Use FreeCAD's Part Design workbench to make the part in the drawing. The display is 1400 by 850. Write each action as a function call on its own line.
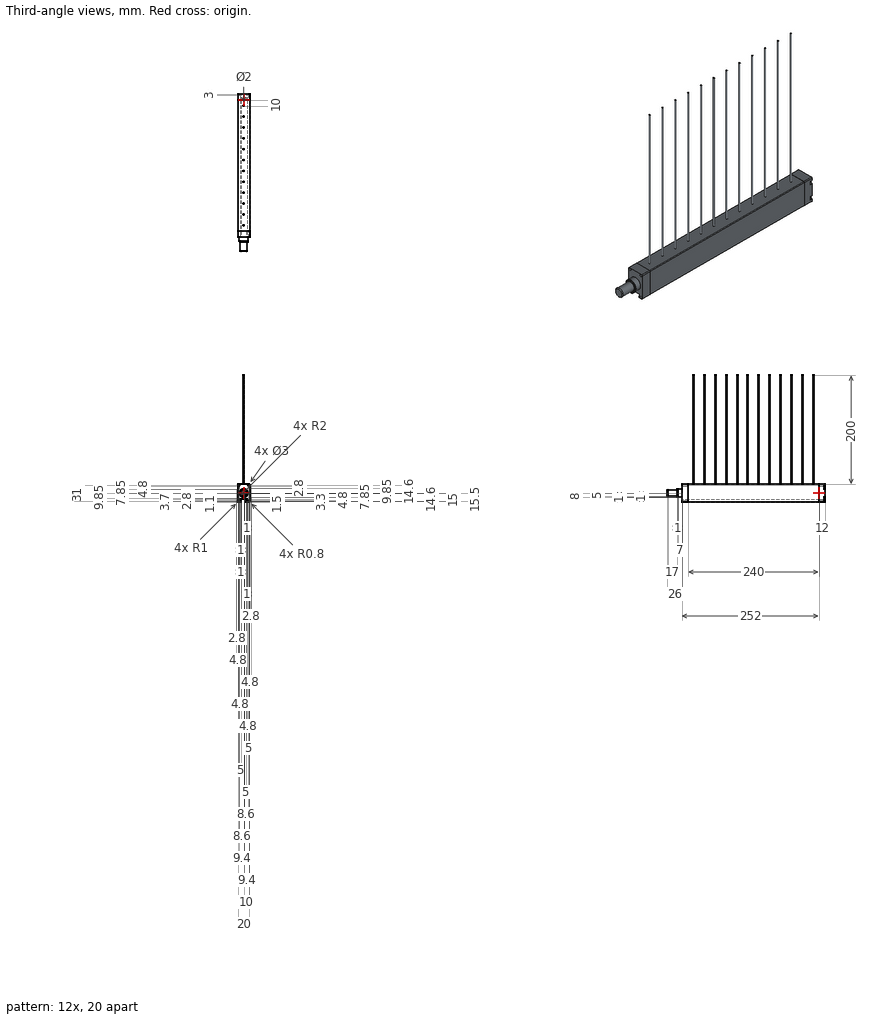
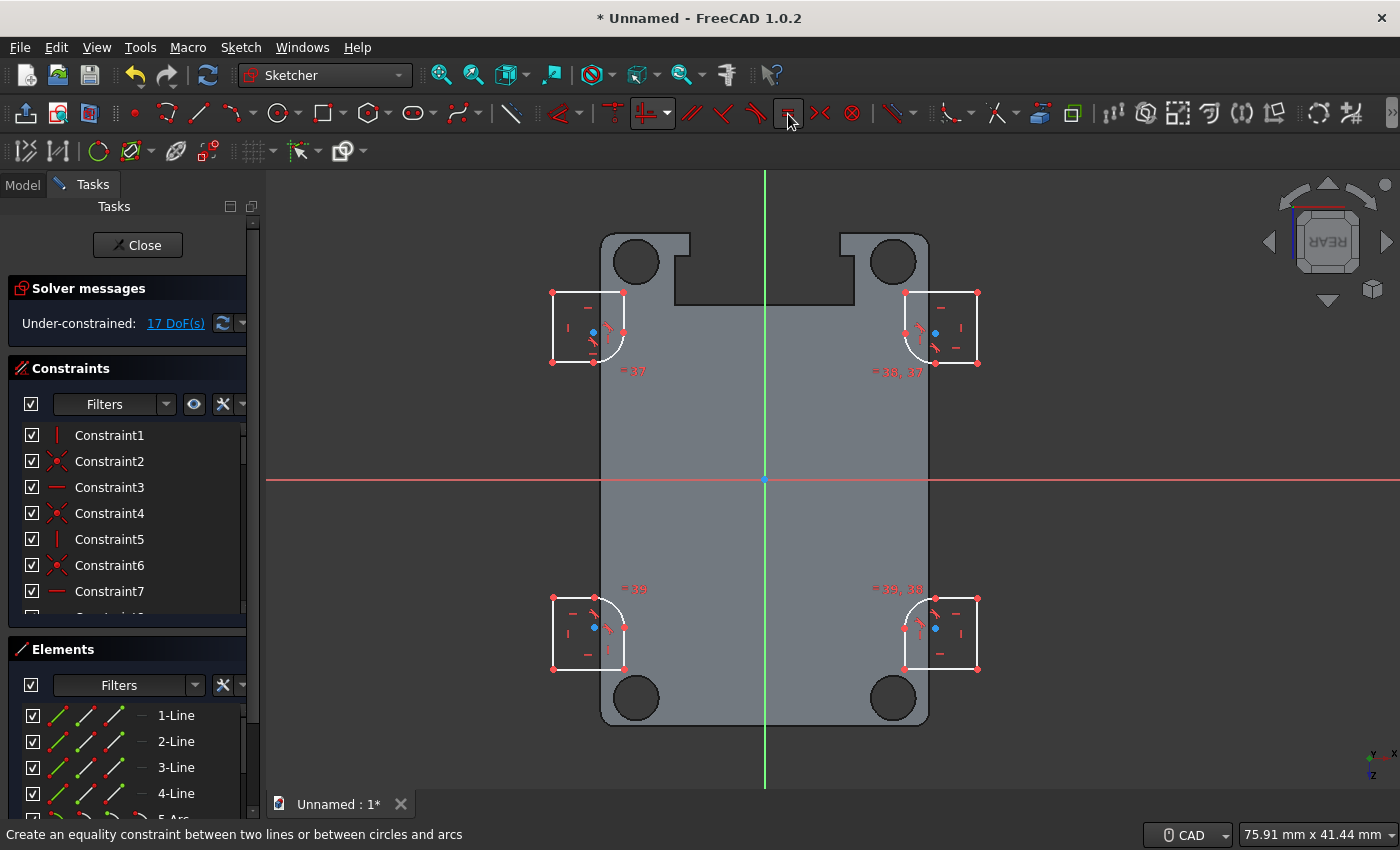
click(558, 114)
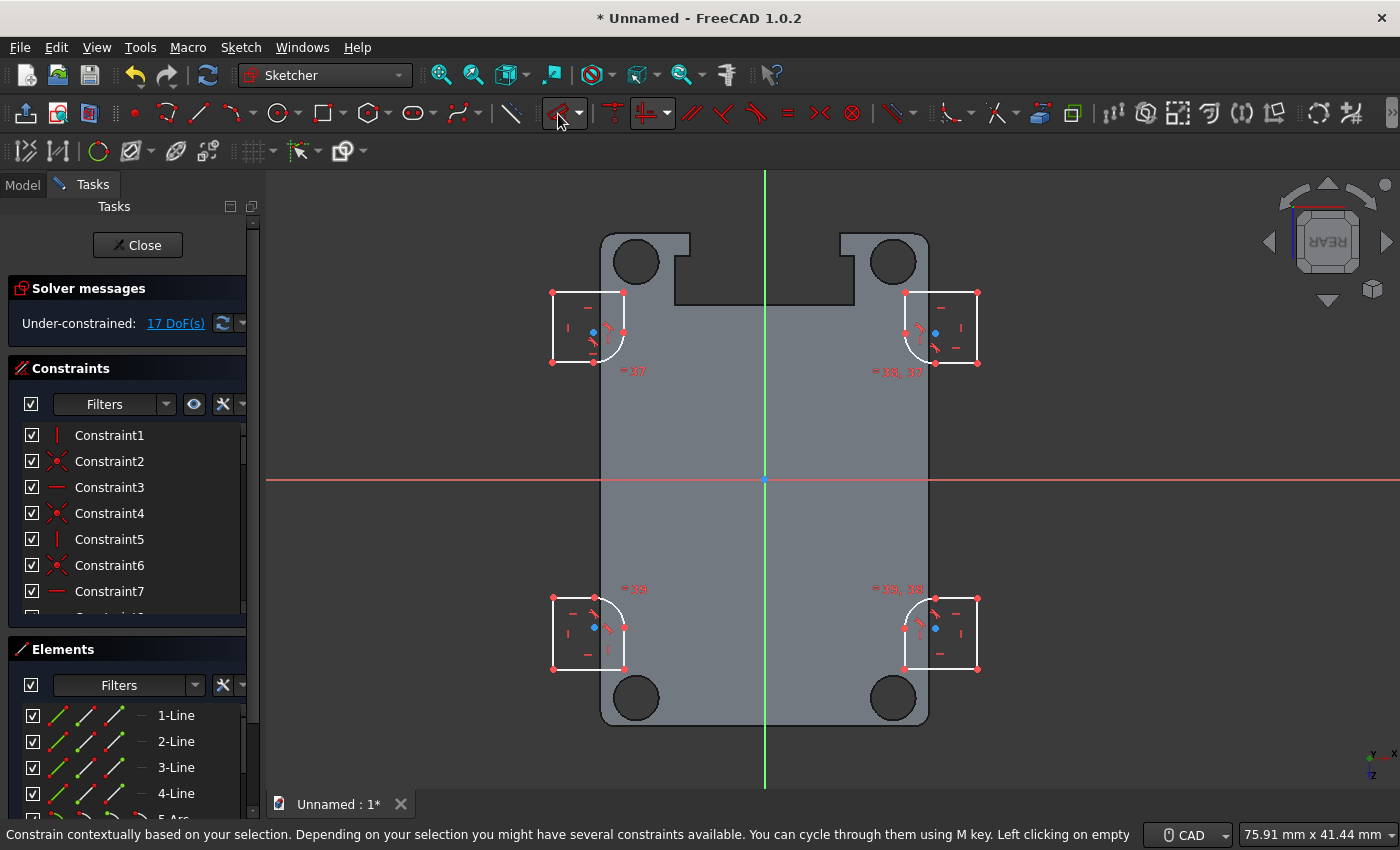
scroll(607, 359, up, 2)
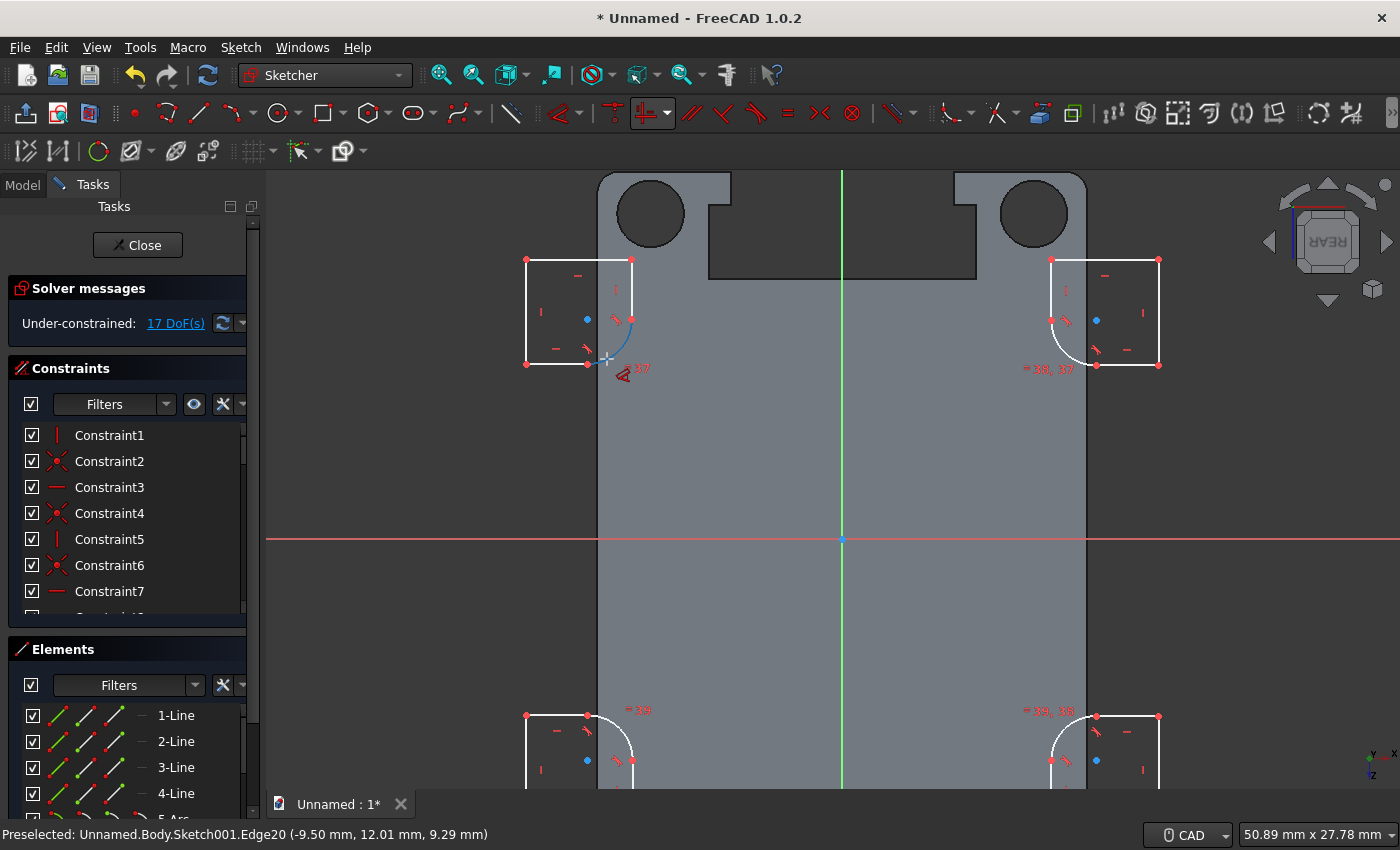
click(607, 359)
click(621, 388)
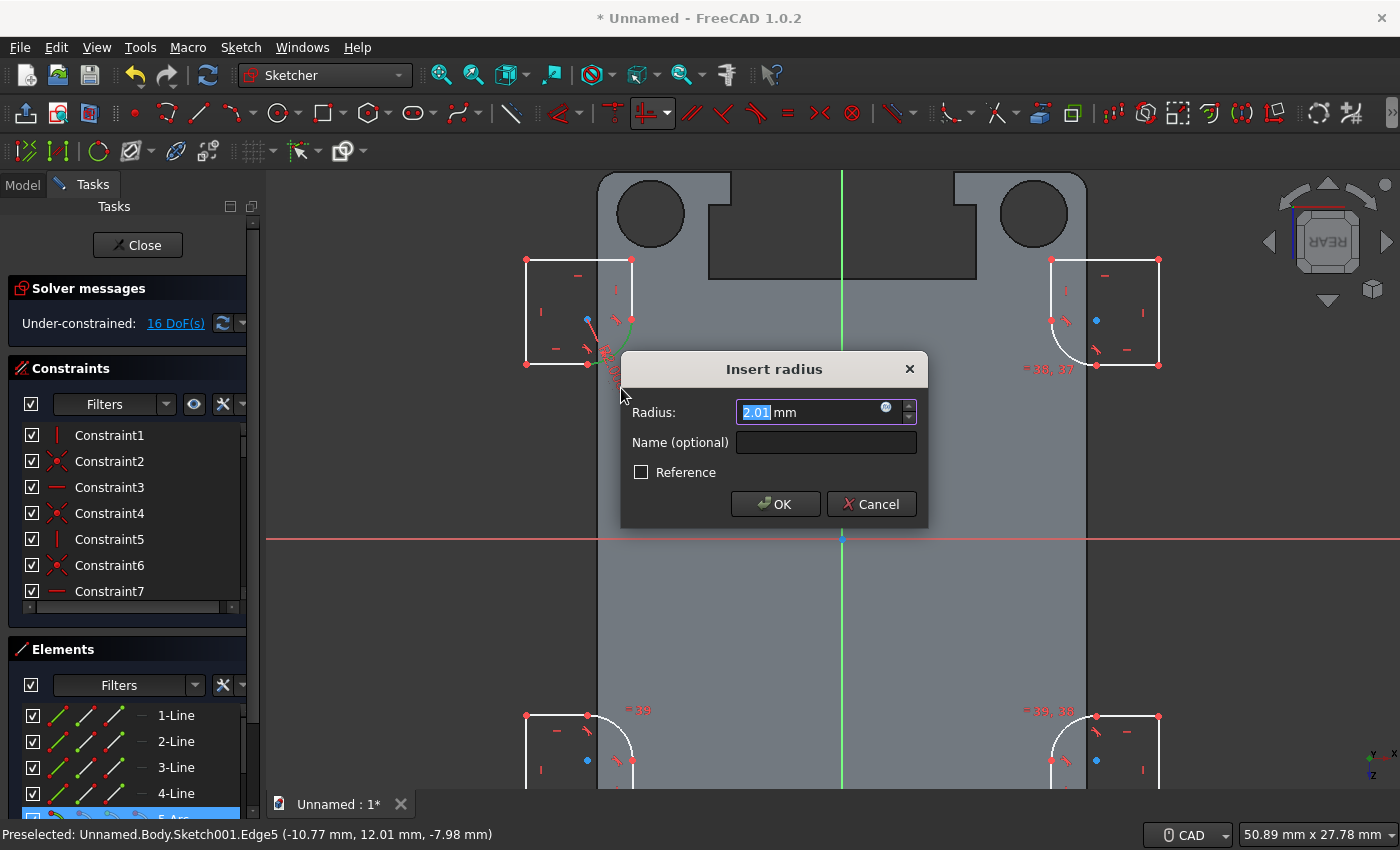
text(2)
key(Return)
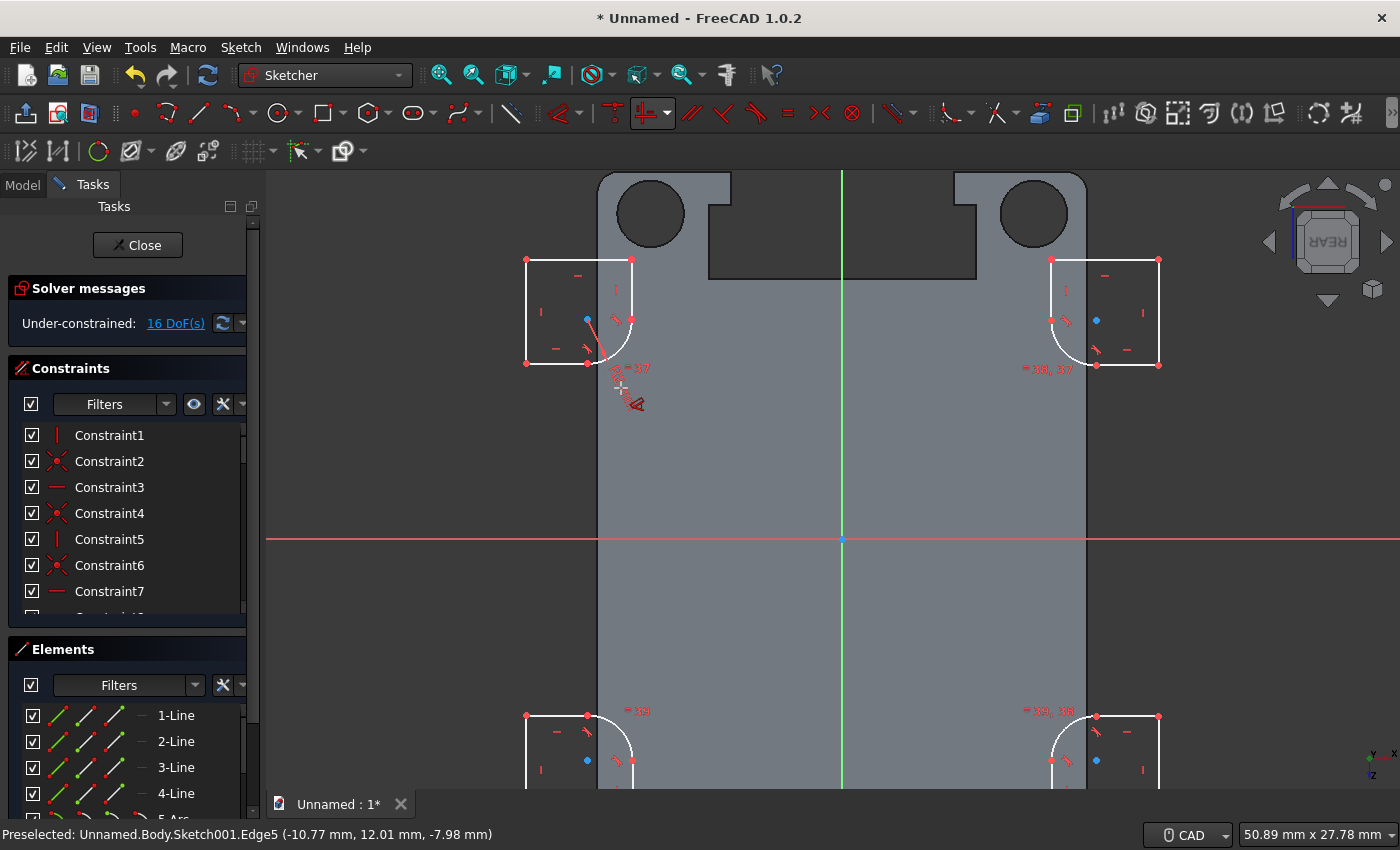
click(632, 301)
click(598, 289)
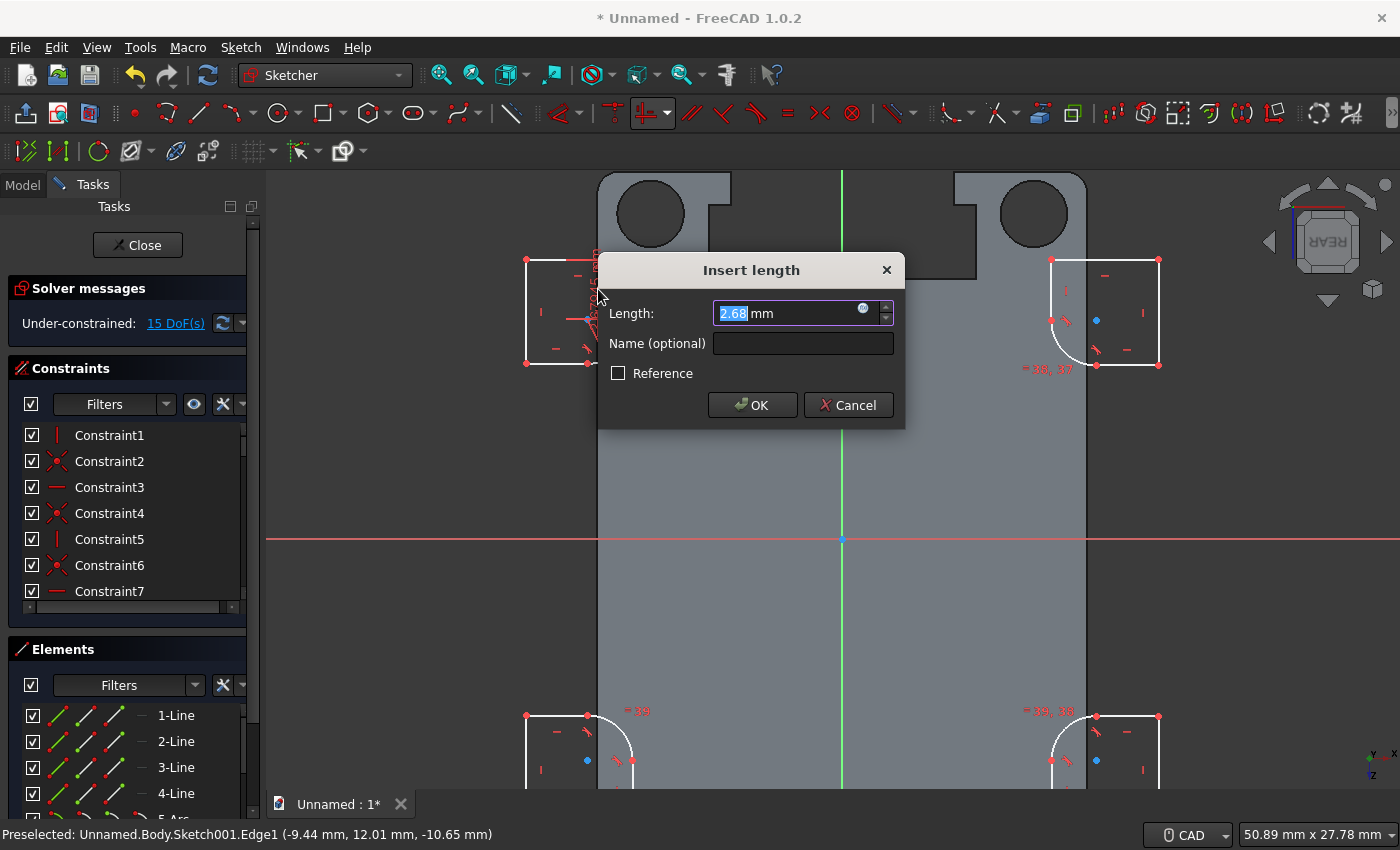
text(2.8)
key(Return)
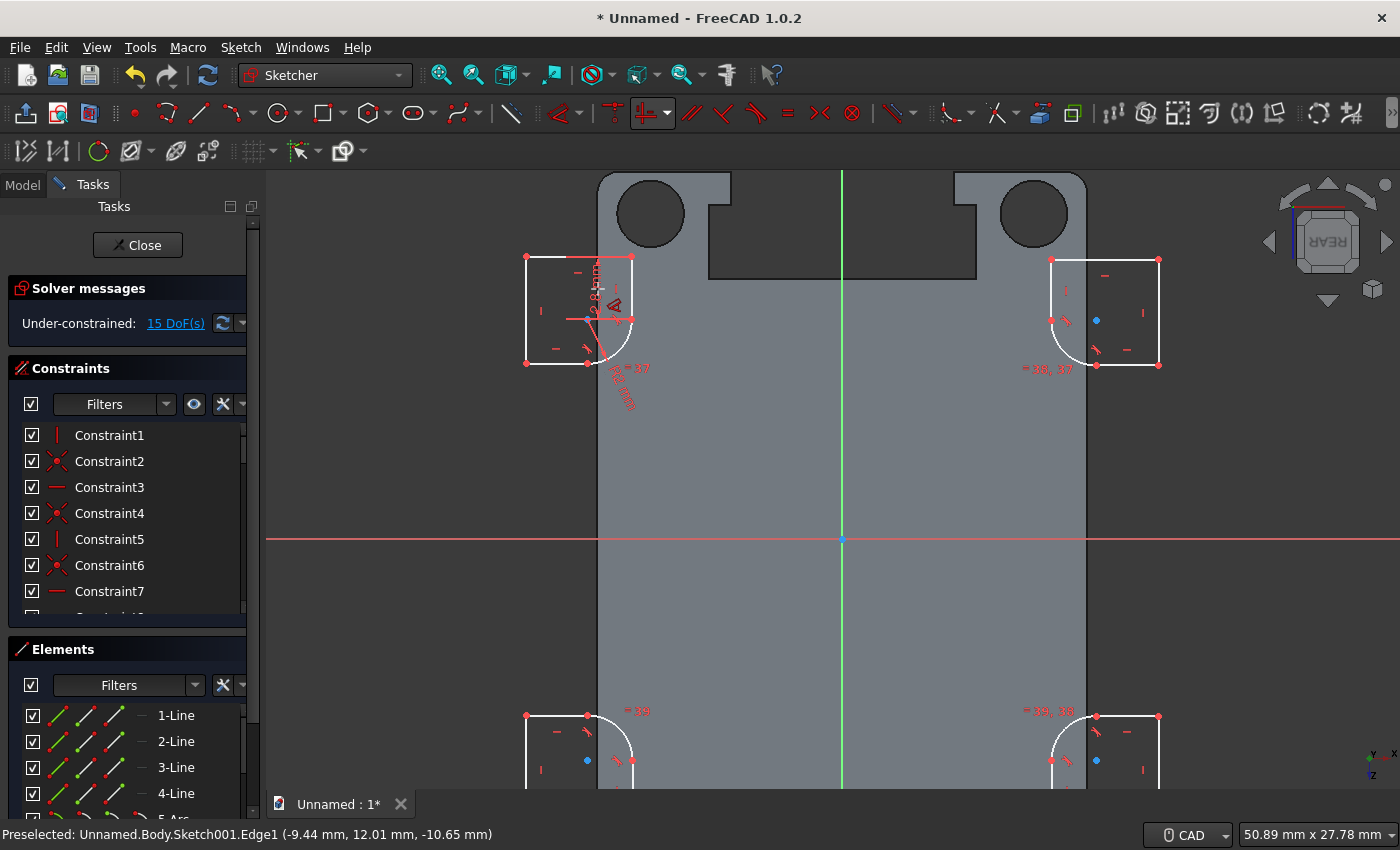
click(600, 257)
click(579, 223)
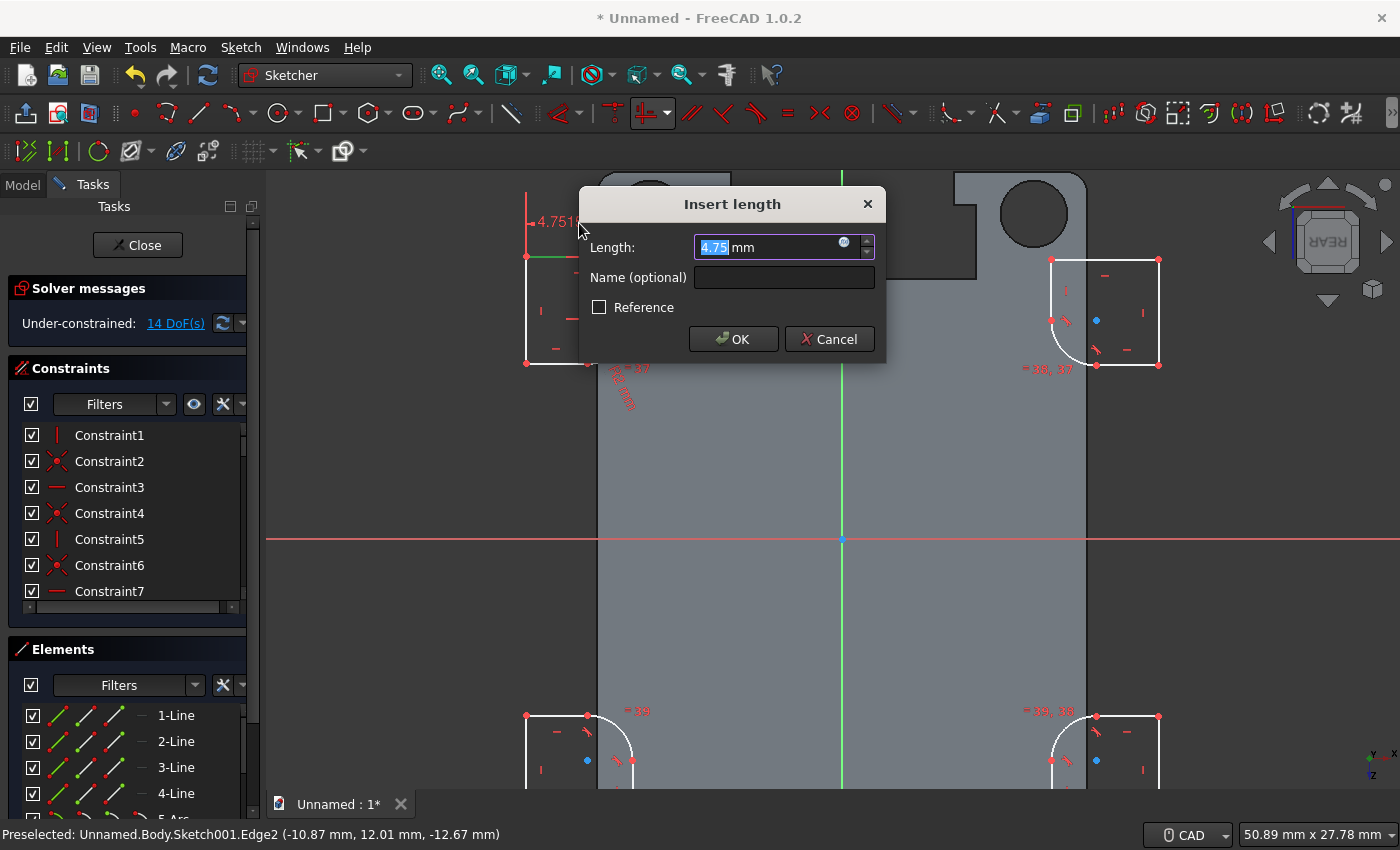
text(4.8)
key(Return)